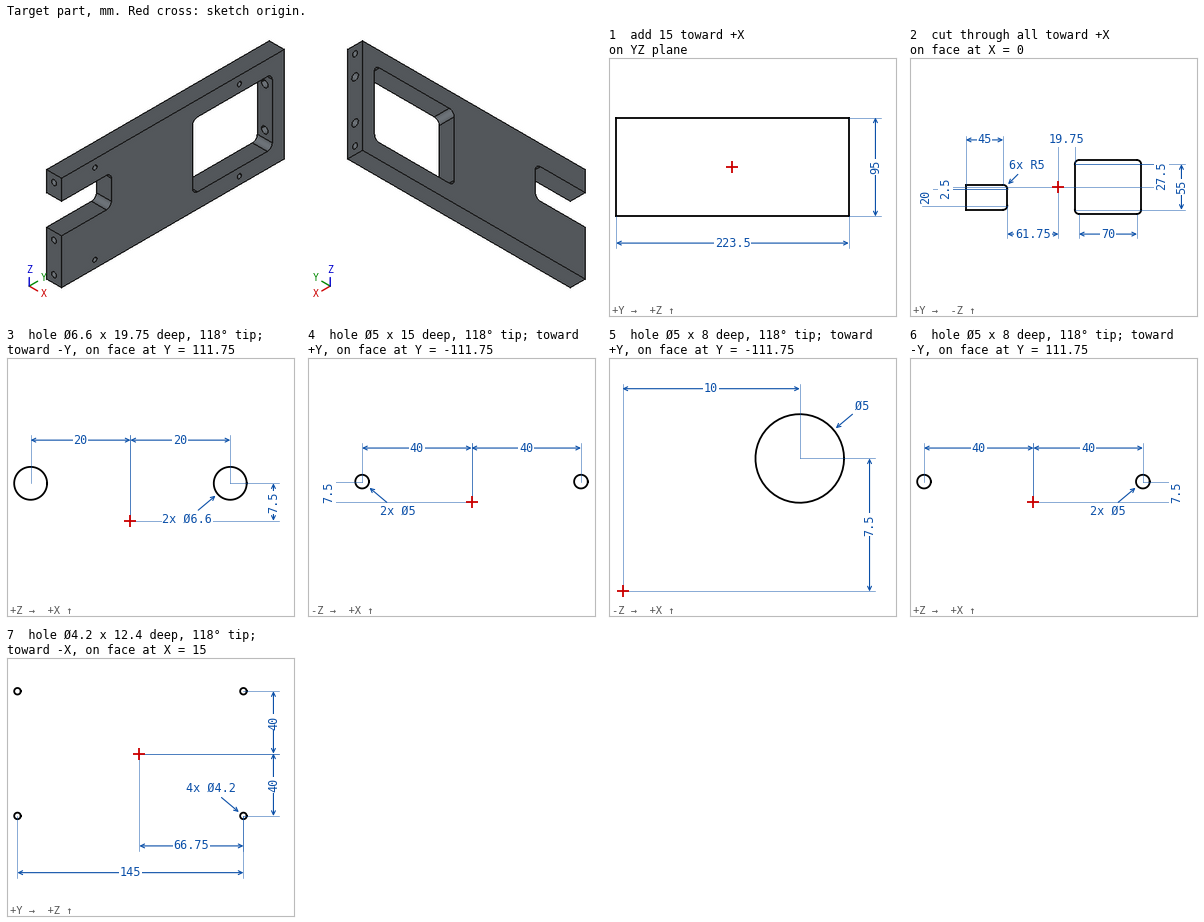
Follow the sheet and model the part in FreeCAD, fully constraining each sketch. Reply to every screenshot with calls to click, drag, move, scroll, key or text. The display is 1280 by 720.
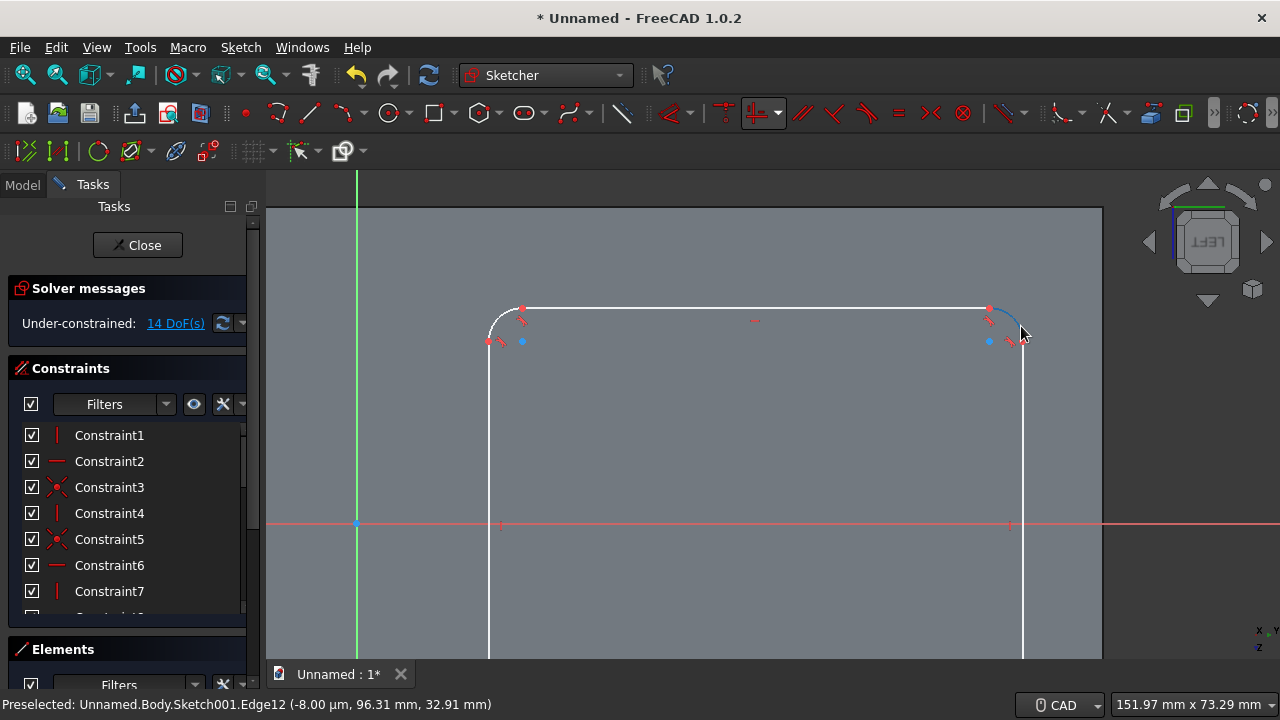
click(1019, 326)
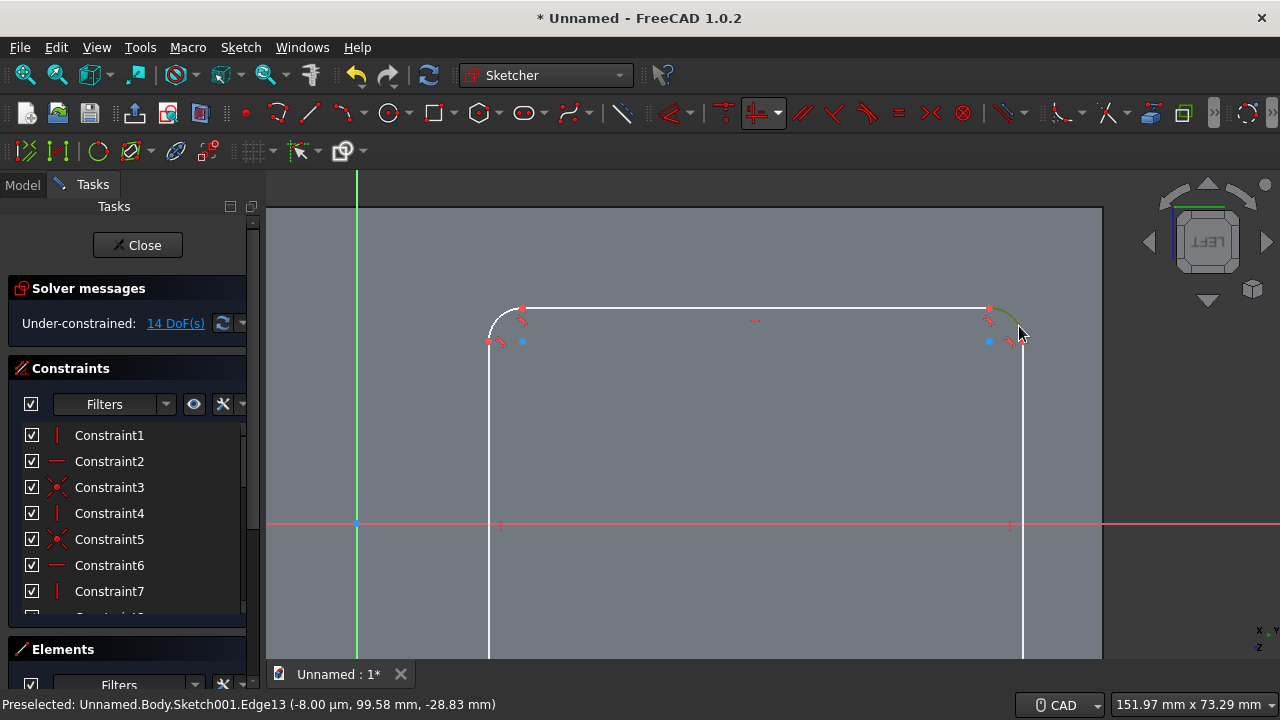
click(507, 312)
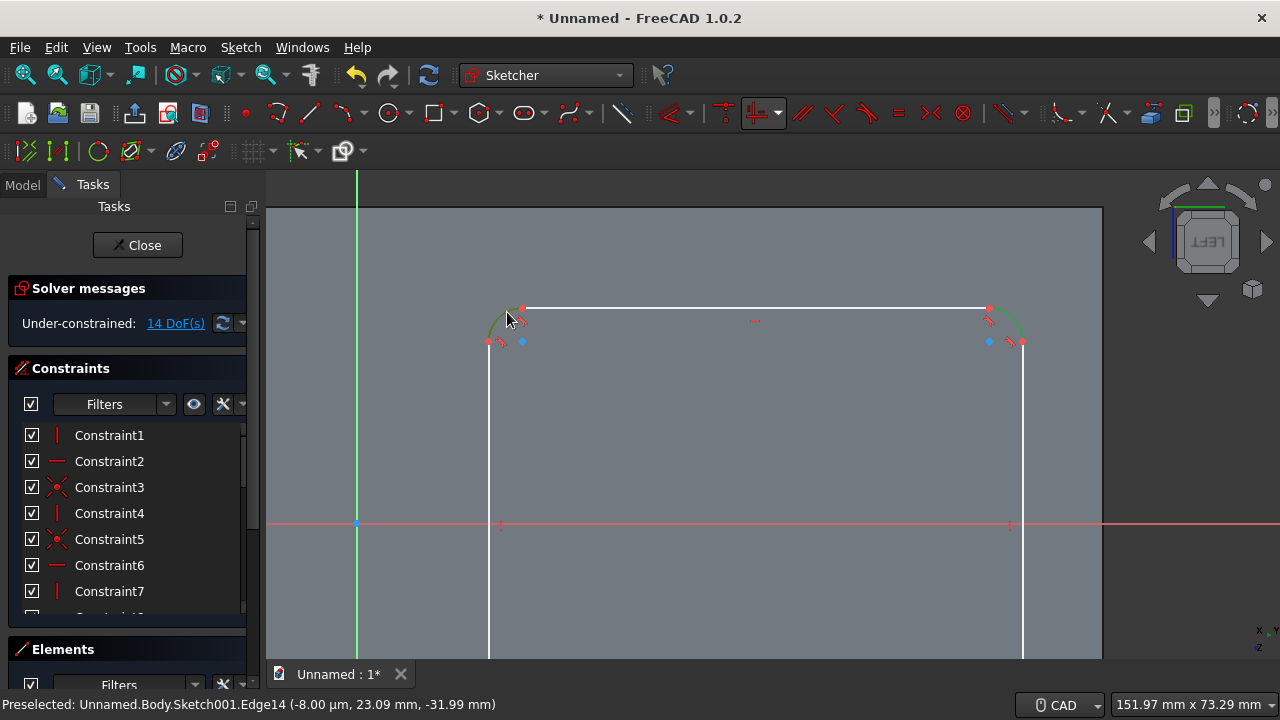
click(900, 114)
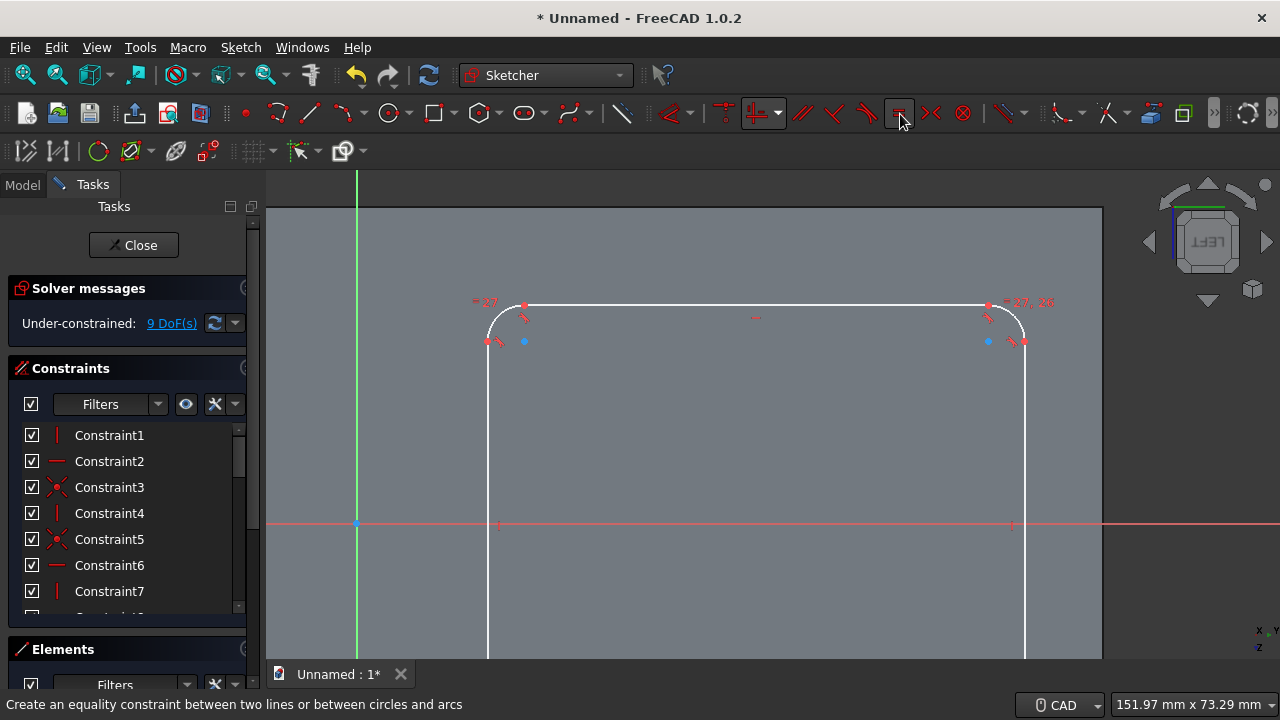
click(670, 114)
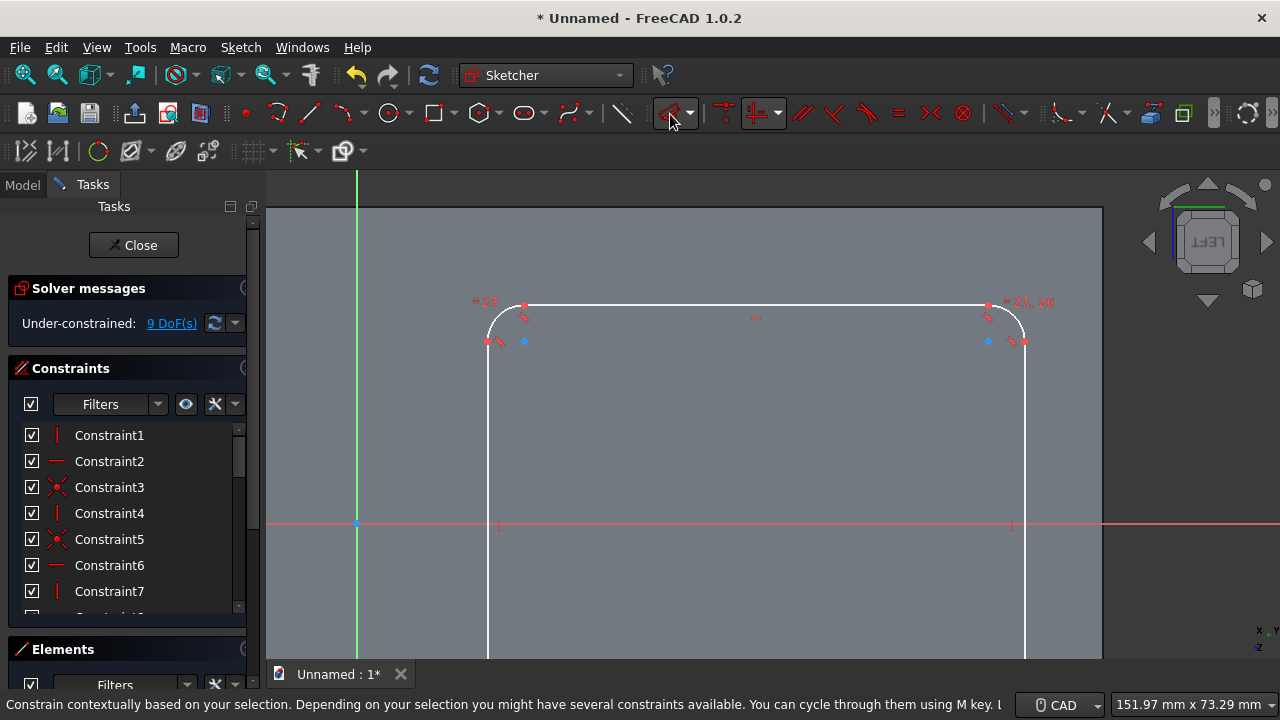
scroll(1021, 325, down, 4)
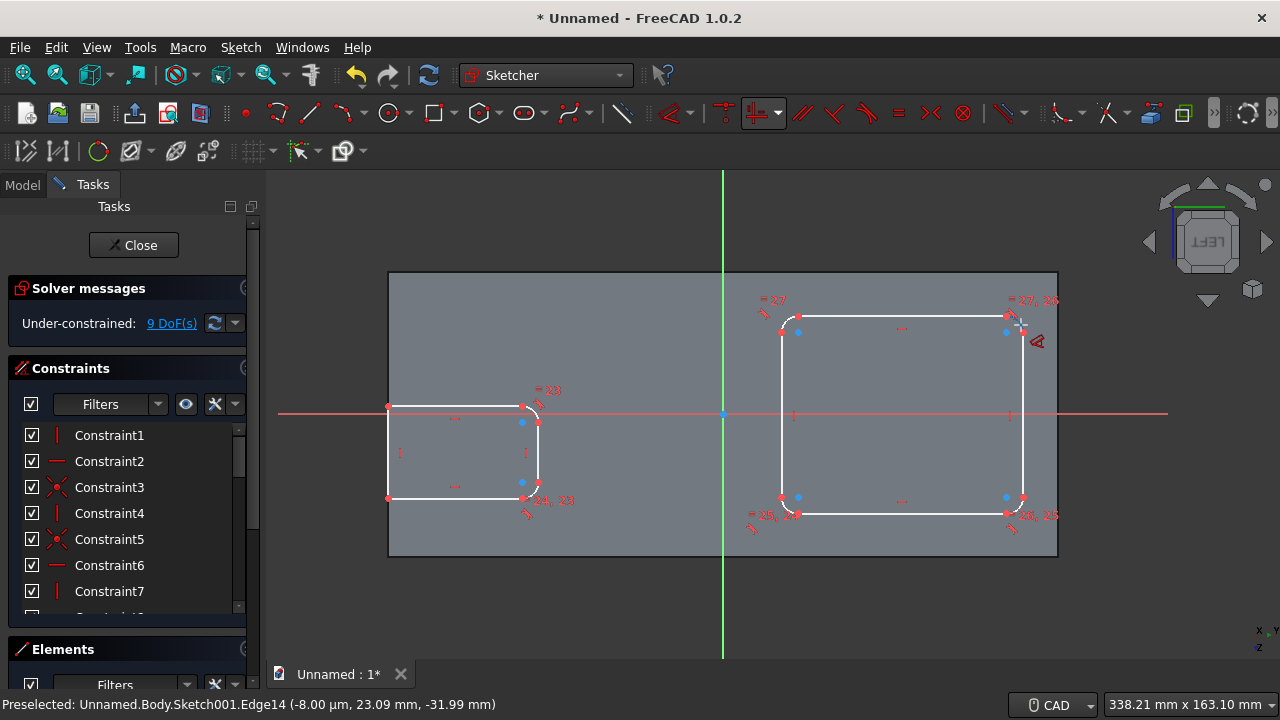
scroll(537, 415, up, 5)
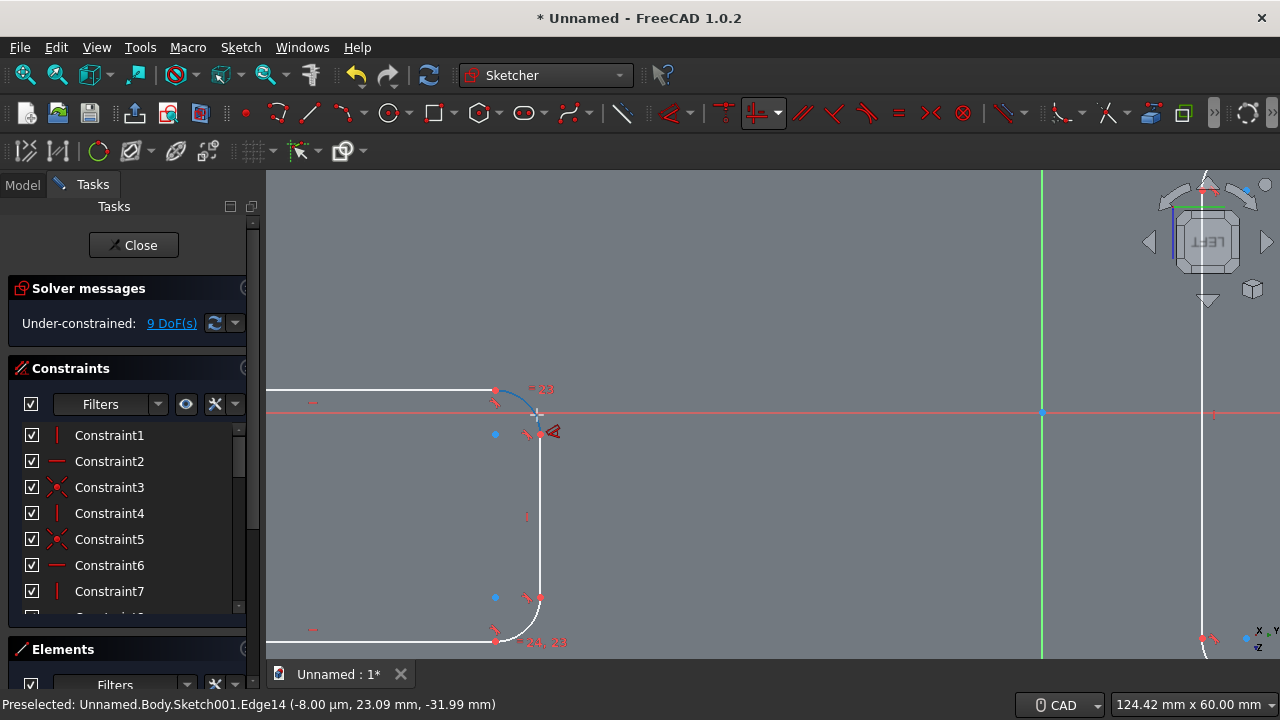
click(535, 415)
click(572, 437)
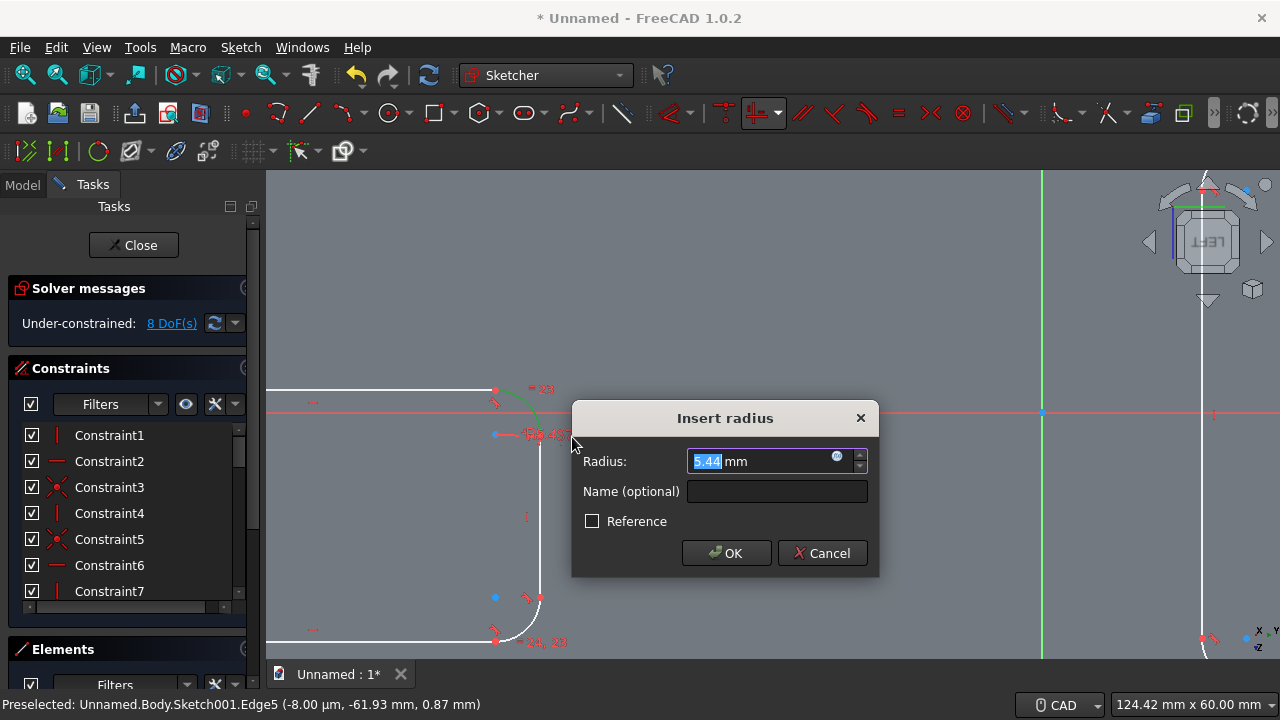
text(5)
key(Return)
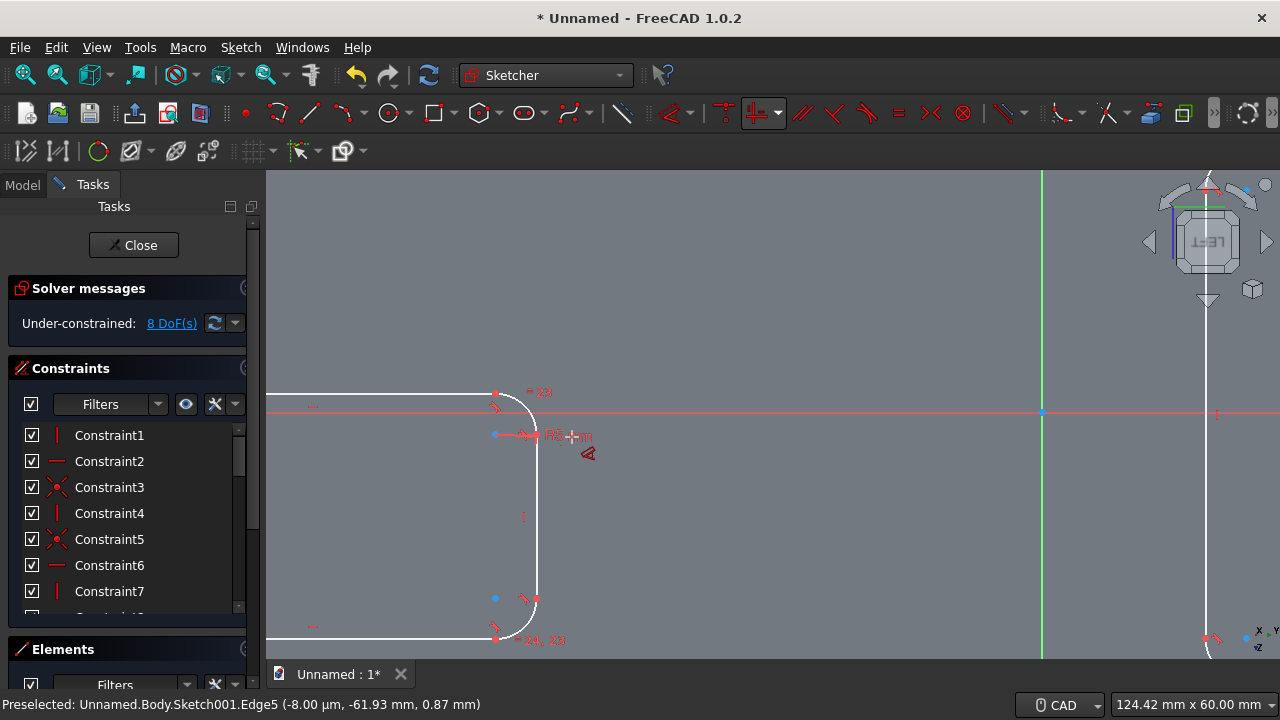
click(537, 549)
click(503, 516)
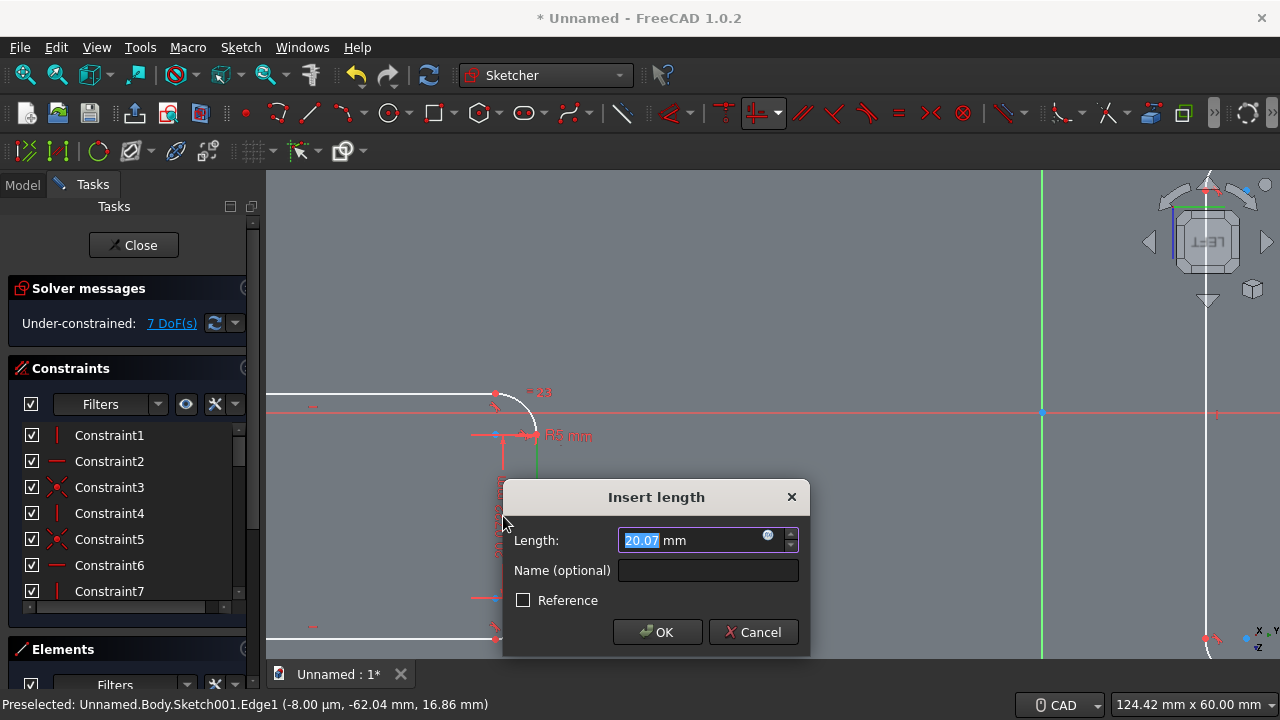
text(20)
key(Return)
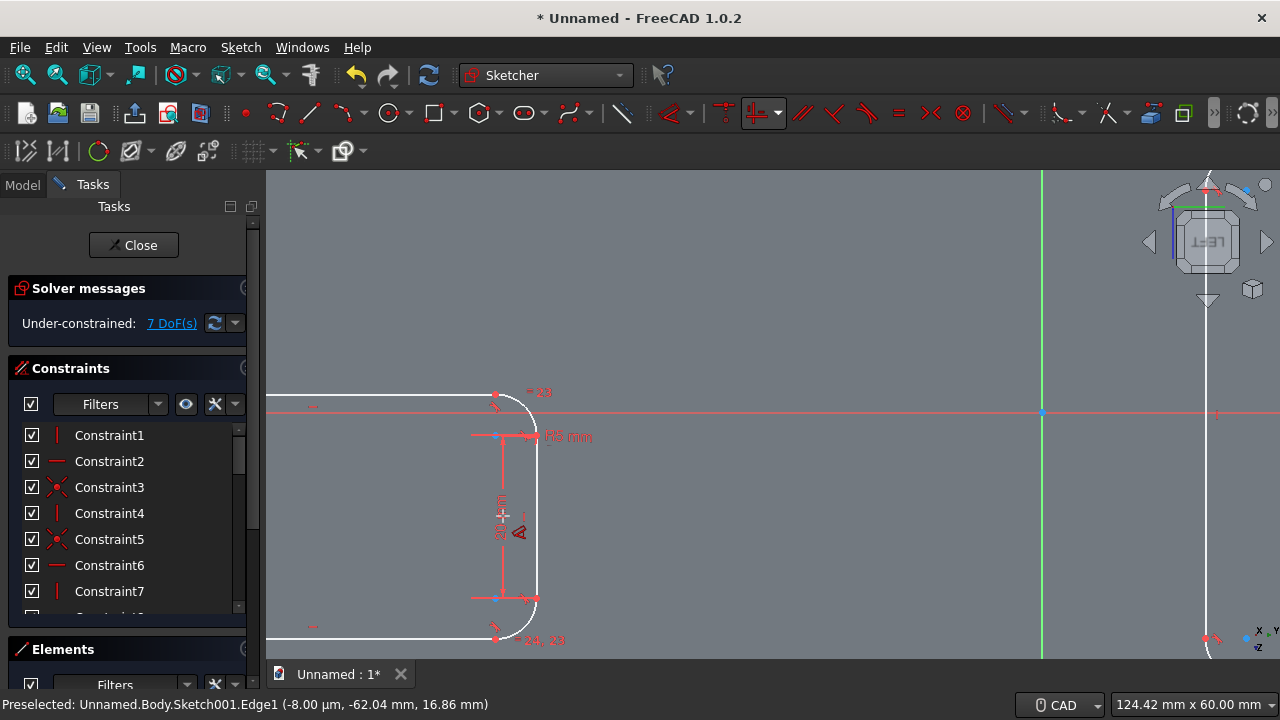
click(387, 395)
click(395, 361)